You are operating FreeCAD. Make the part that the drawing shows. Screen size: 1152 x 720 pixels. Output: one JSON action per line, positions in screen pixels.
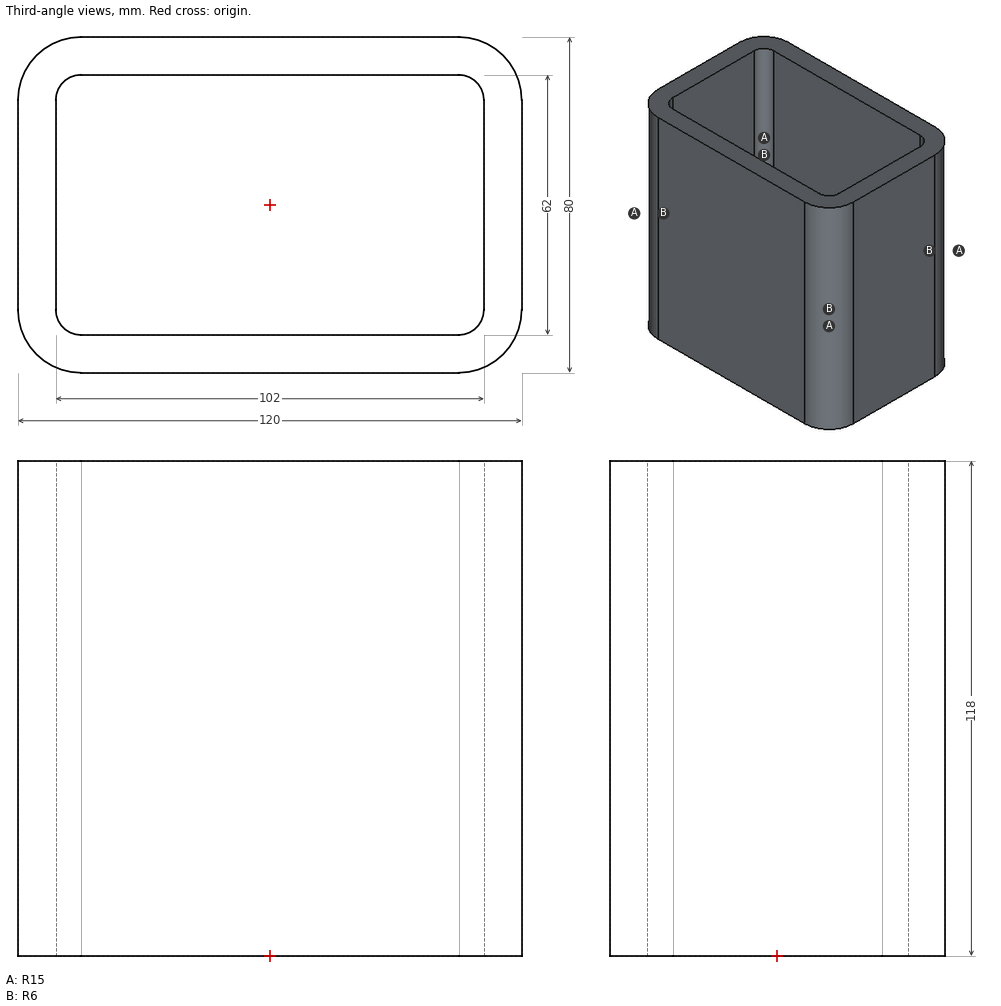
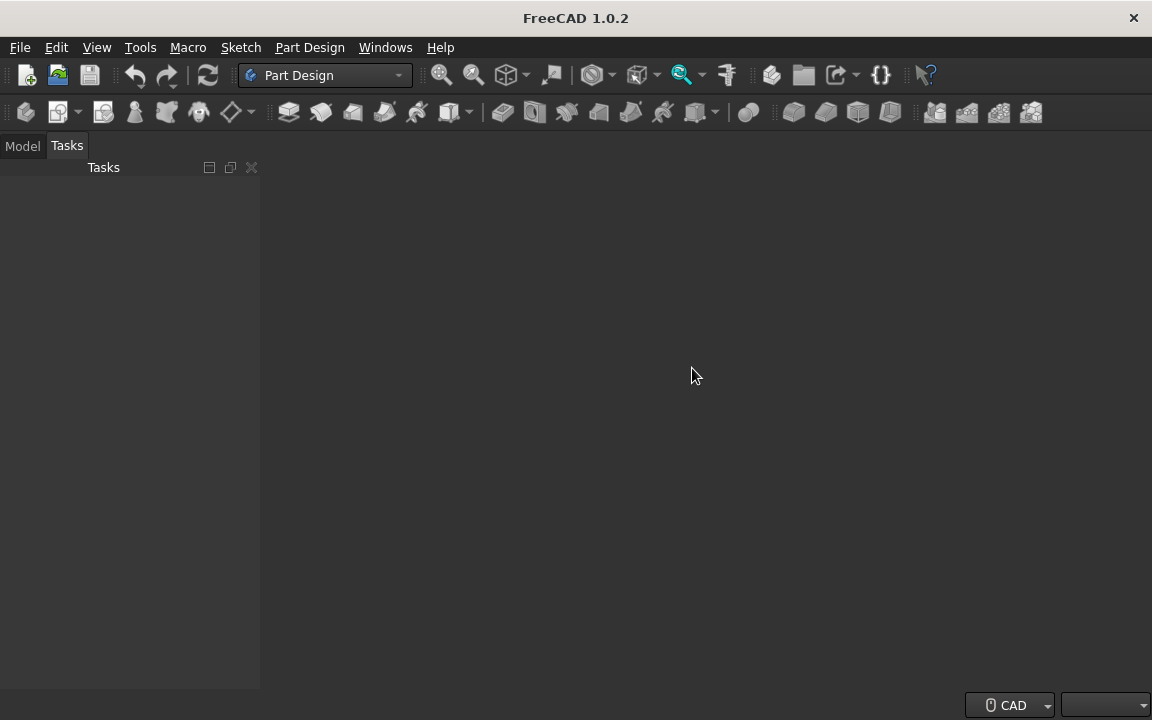
{"action": "left_click", "coordinate": [26, 76]}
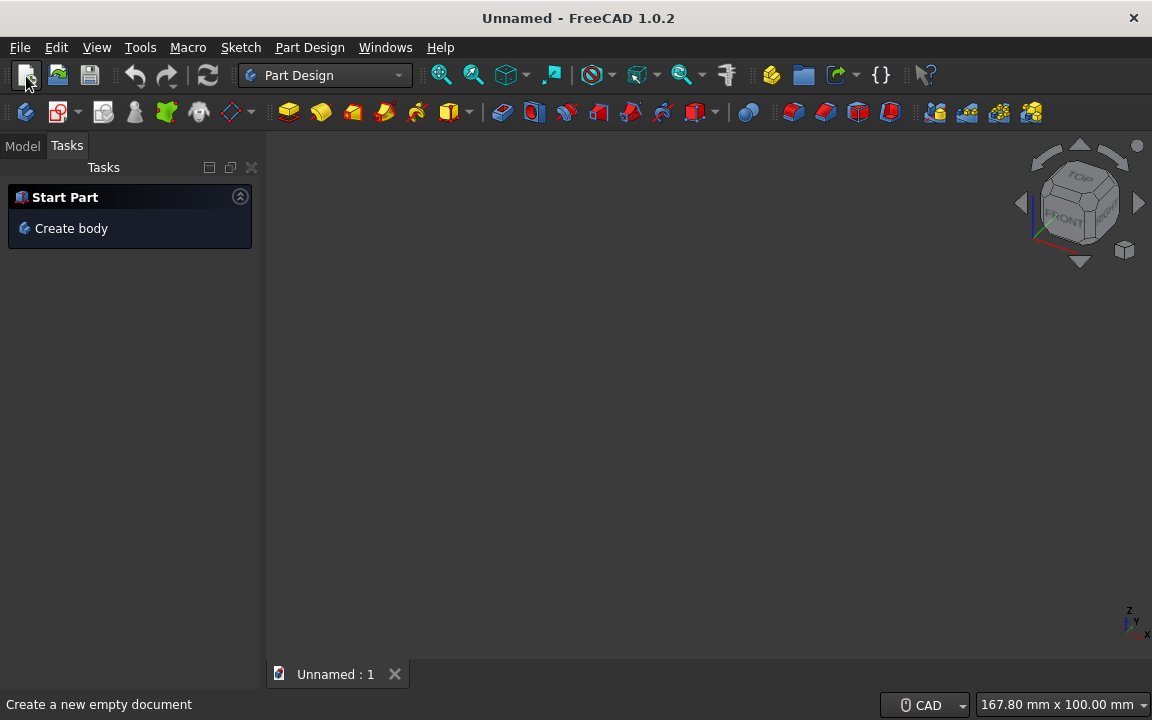
{"action": "left_click", "coordinate": [58, 112]}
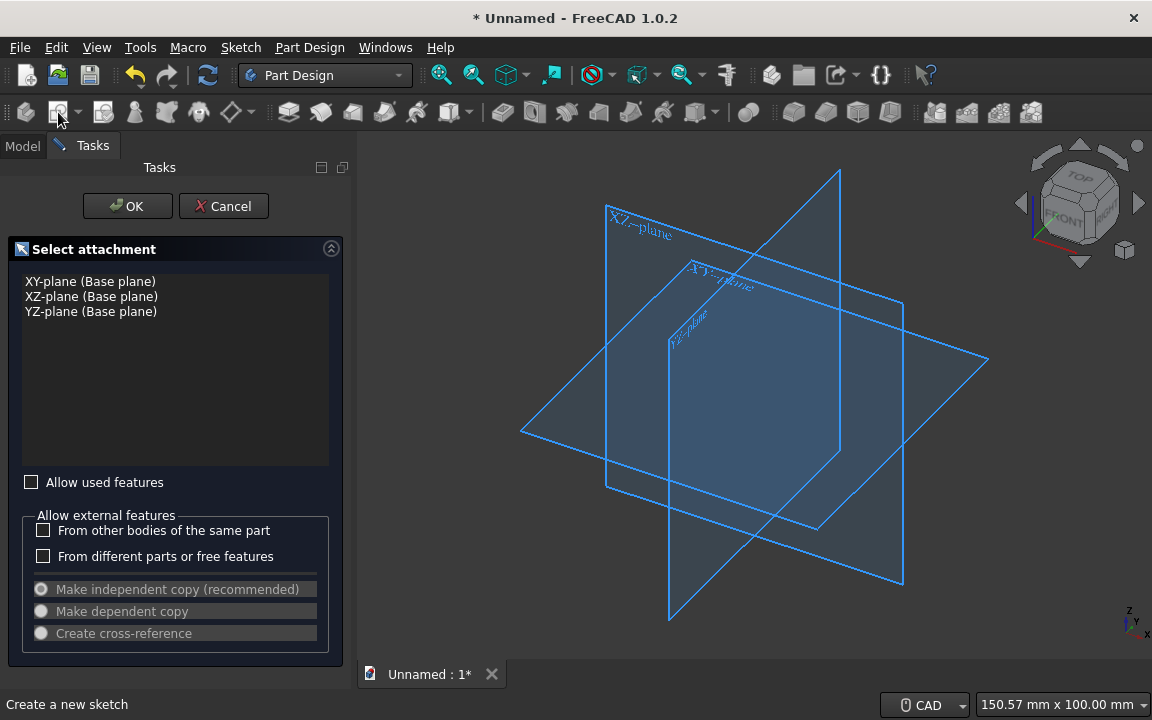
{"action": "left_click", "coordinate": [82, 282]}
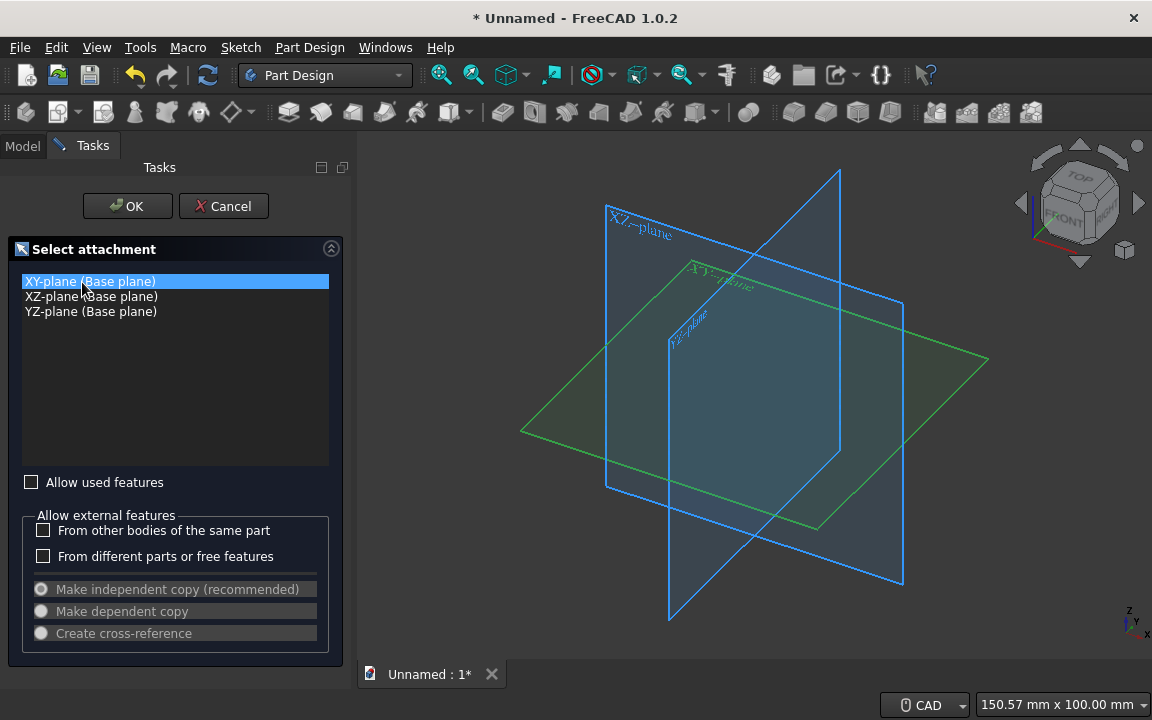
{"action": "left_click", "coordinate": [128, 206]}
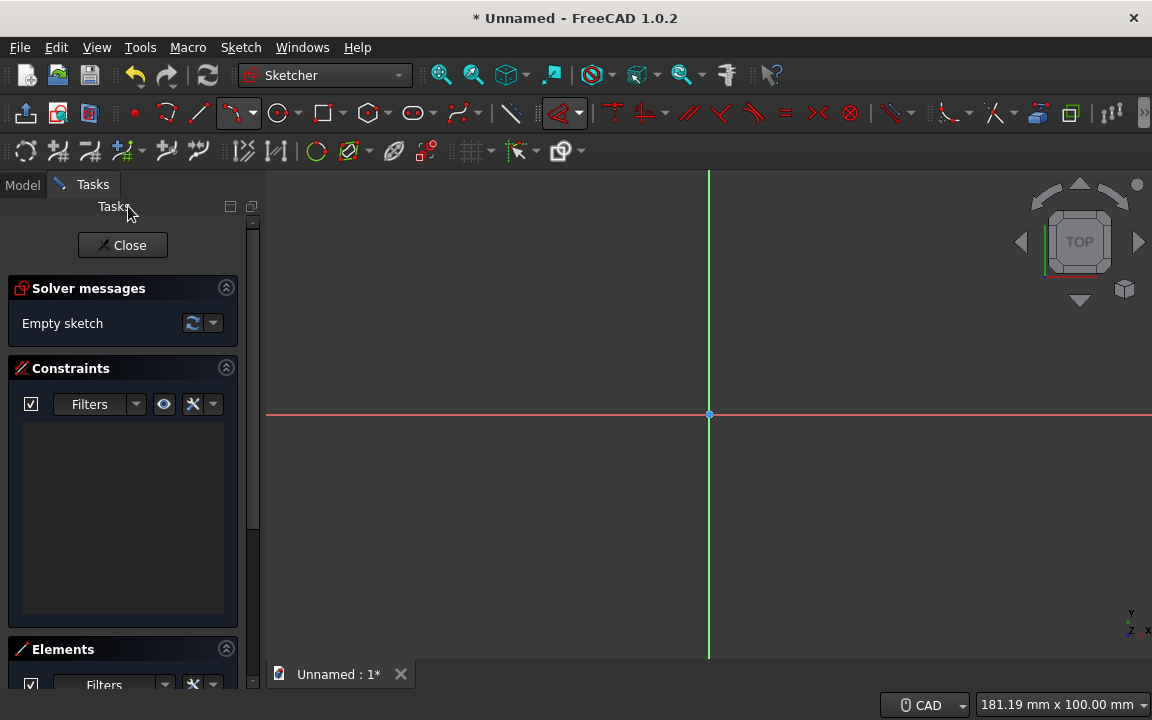
{"action": "scroll", "coordinate": [331, 415], "scroll_direction": "down", "scroll_amount": 1}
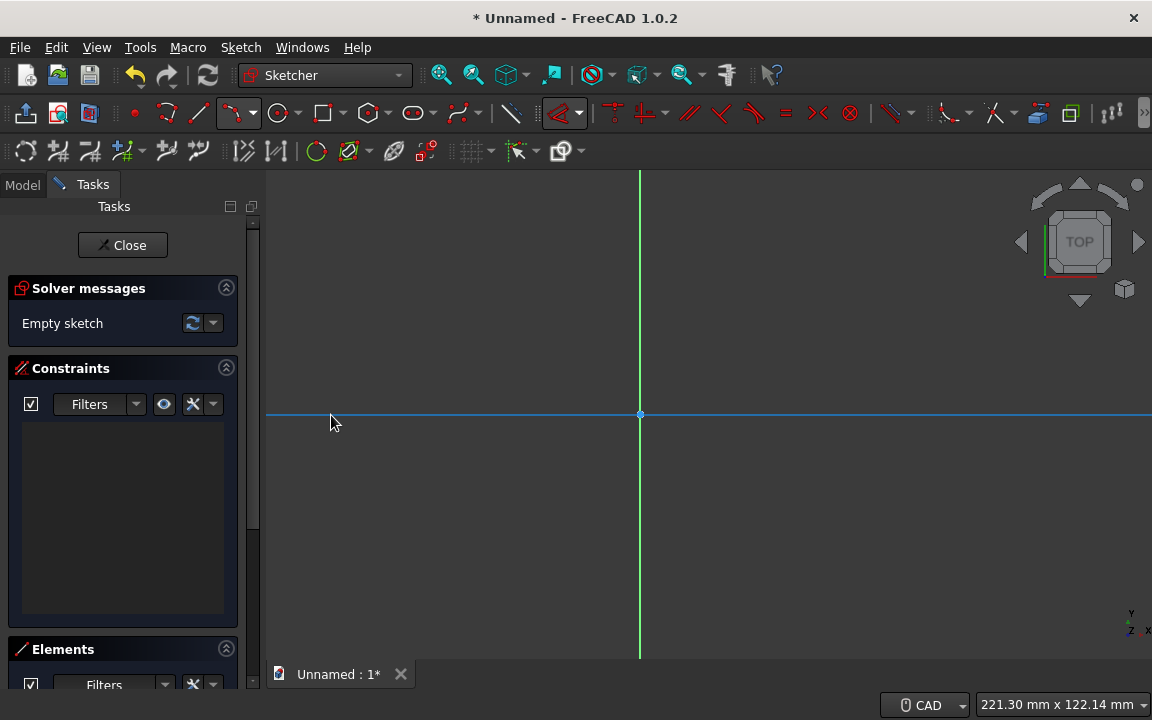
{"action": "left_click", "coordinate": [346, 114]}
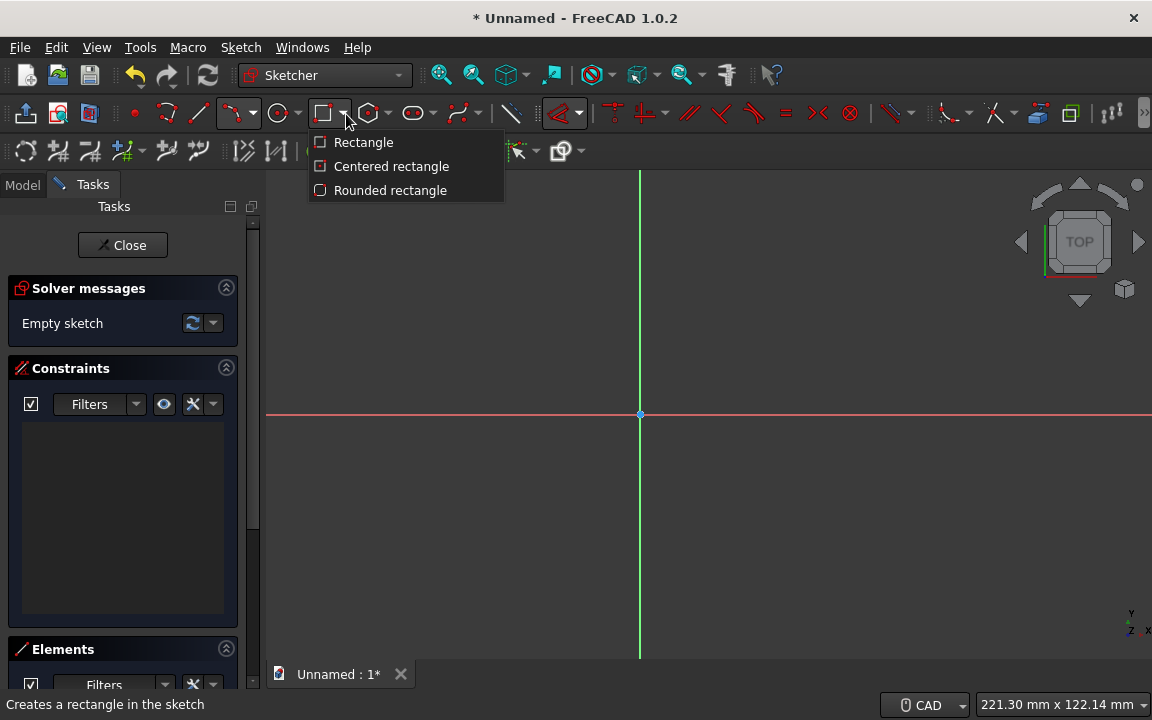
{"action": "left_click", "coordinate": [406, 166]}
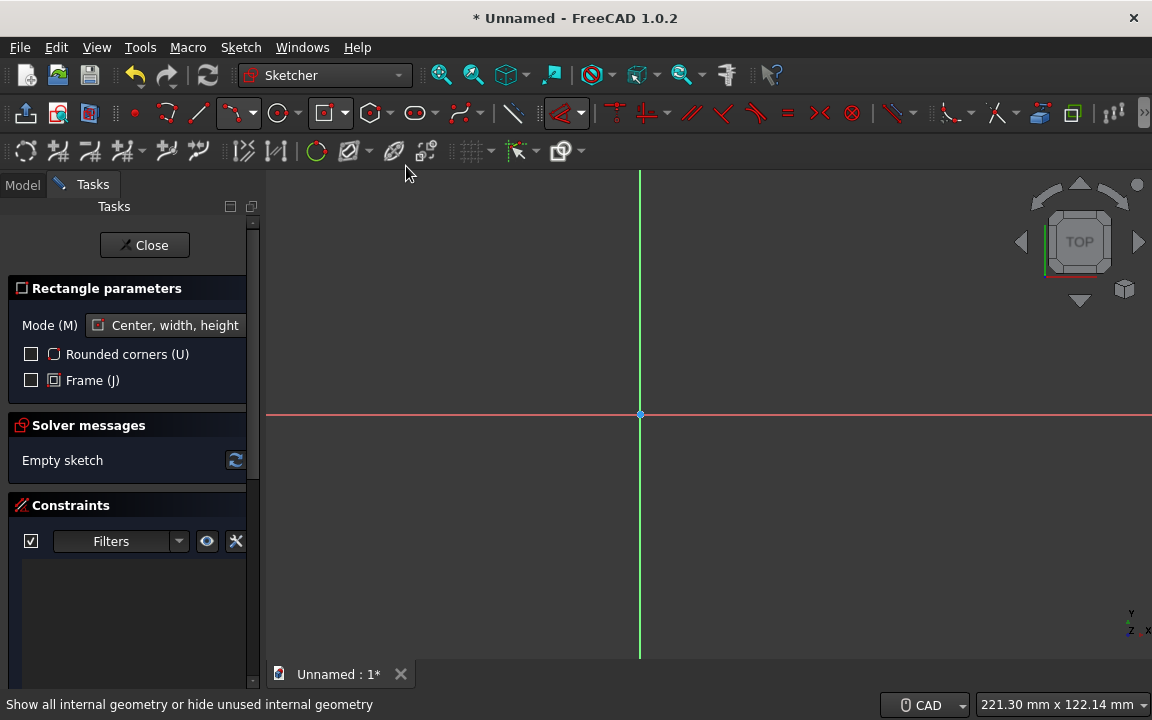
{"action": "left_click", "coordinate": [640, 415]}
{"action": "mouse_move", "coordinate": [881, 255]}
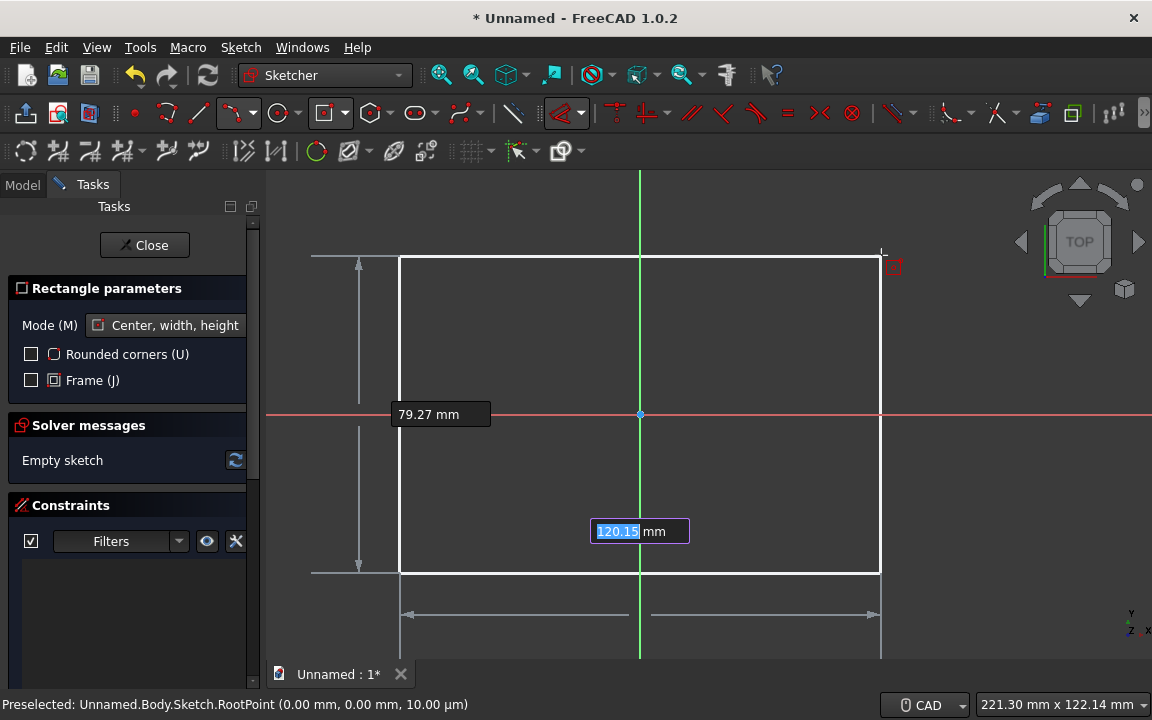
{"action": "type", "text": "120"}
{"action": "key", "text": "Tab"}
{"action": "type", "text": "80"}
{"action": "key", "text": "Return"}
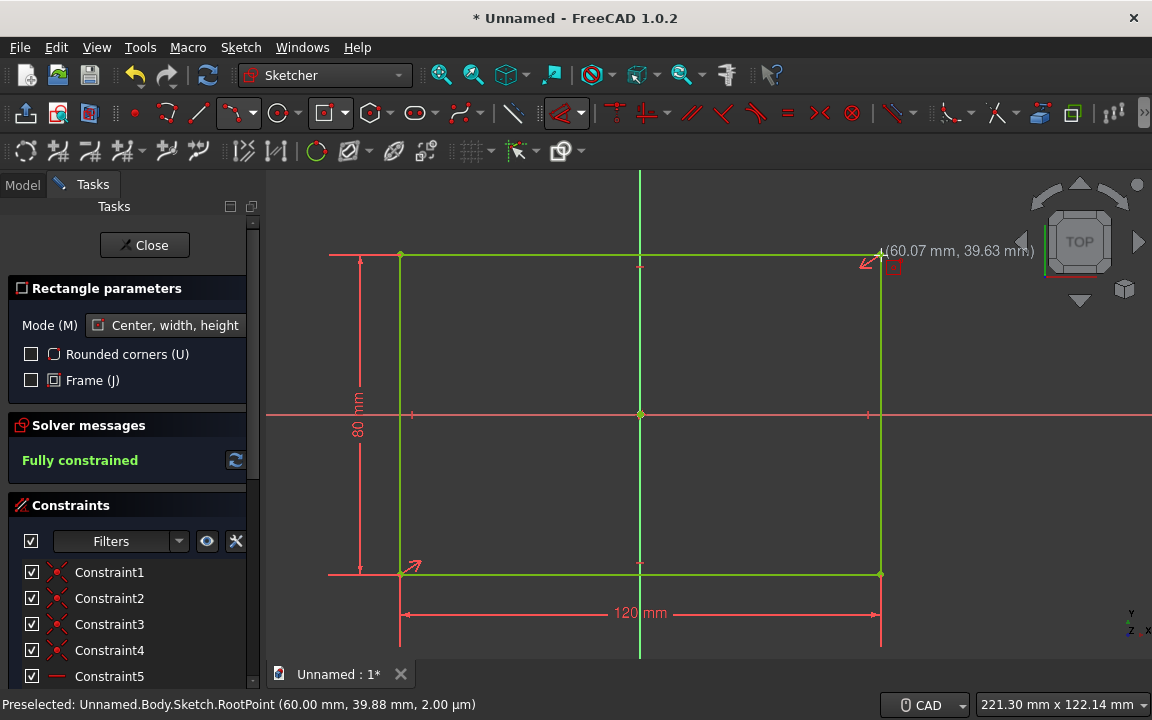
{"action": "left_click", "coordinate": [640, 415]}
{"action": "mouse_move", "coordinate": [845, 291]}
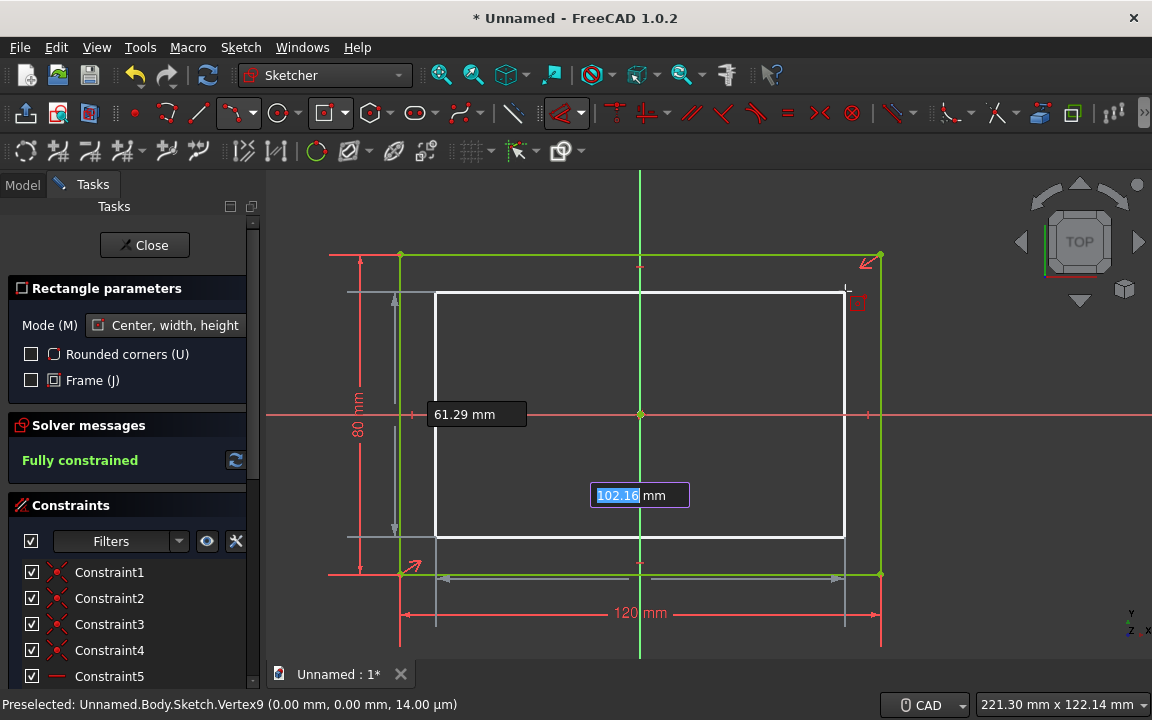
{"action": "type", "text": "102"}
{"action": "key", "text": "Tab"}
{"action": "type", "text": "62"}
{"action": "key", "text": "Return"}
{"action": "key", "text": "Escape"}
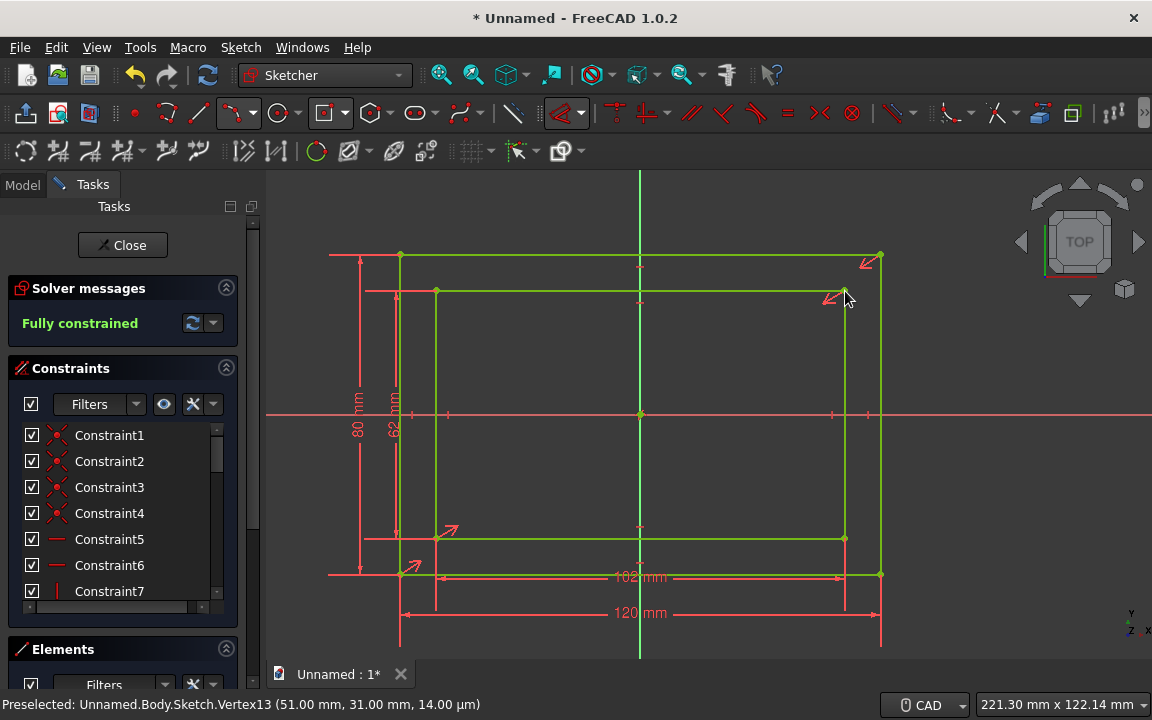
{"action": "left_click", "coordinate": [123, 245]}